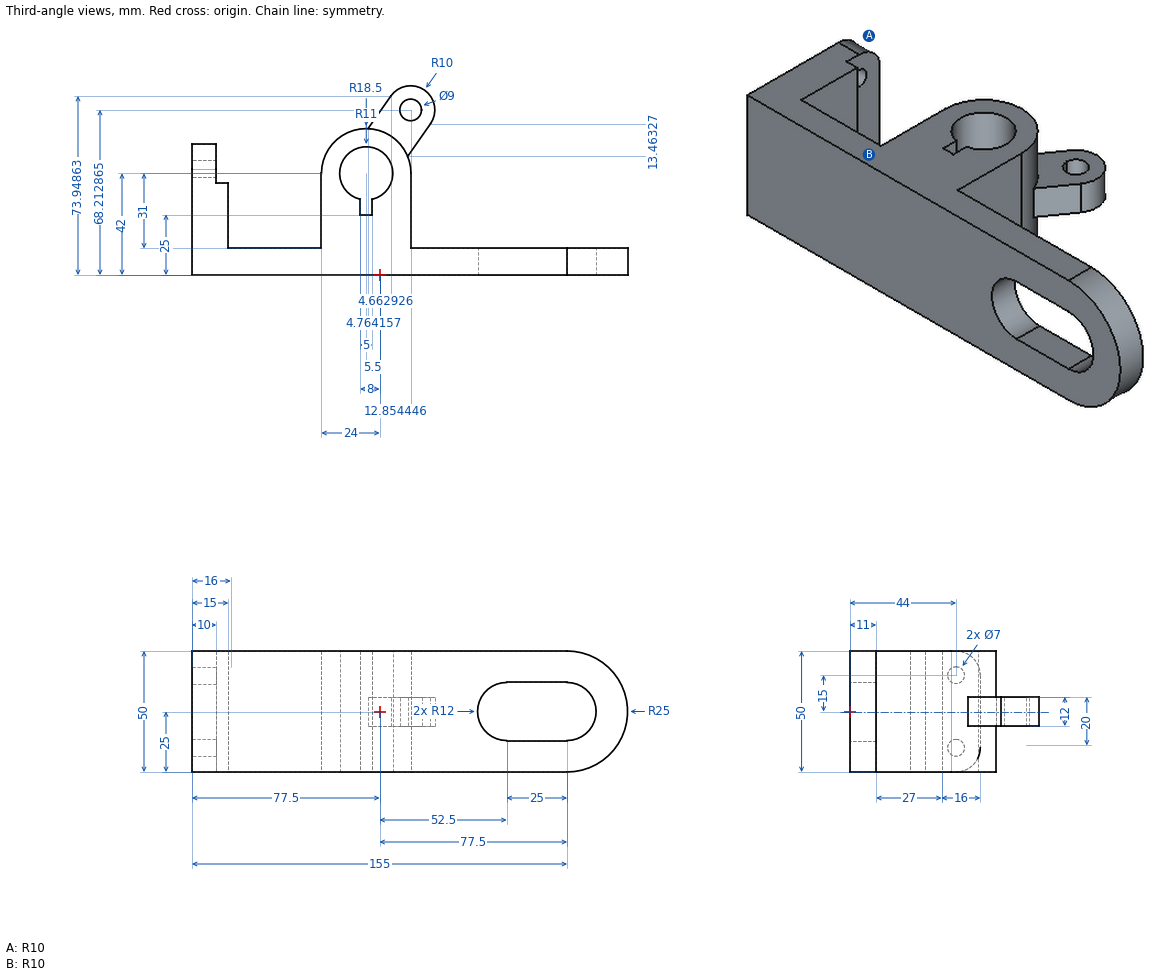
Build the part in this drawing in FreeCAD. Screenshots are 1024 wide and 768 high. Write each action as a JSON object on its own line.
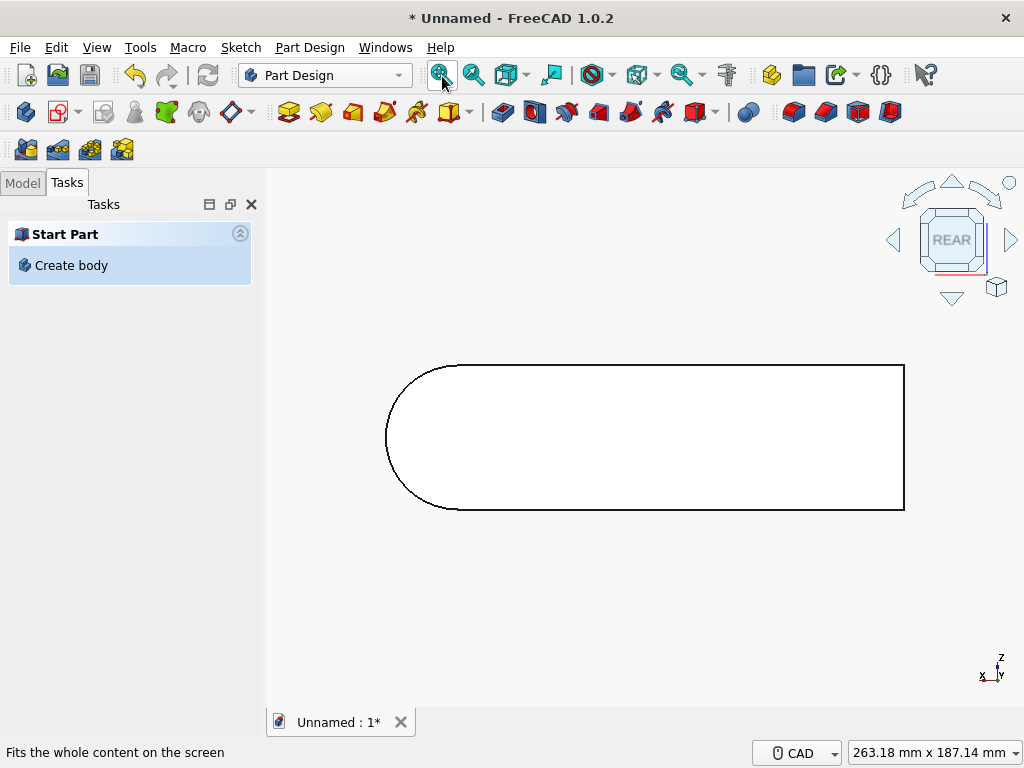
{"action": "left_click", "coordinate": [497, 436]}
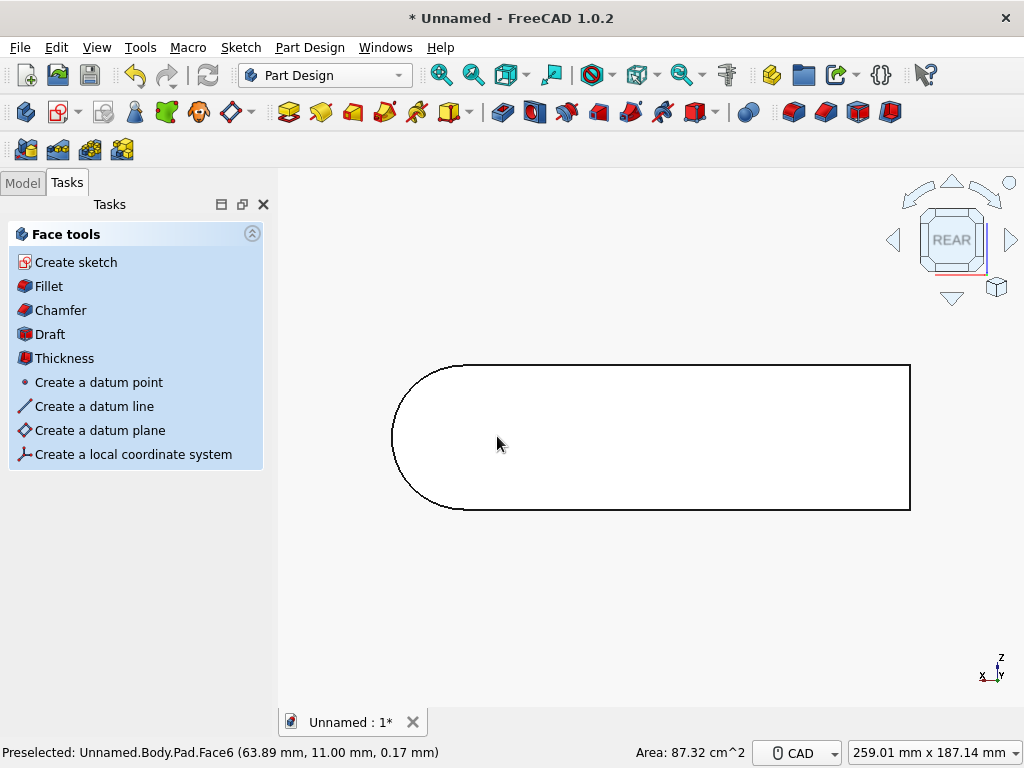
{"action": "left_click", "coordinate": [58, 112]}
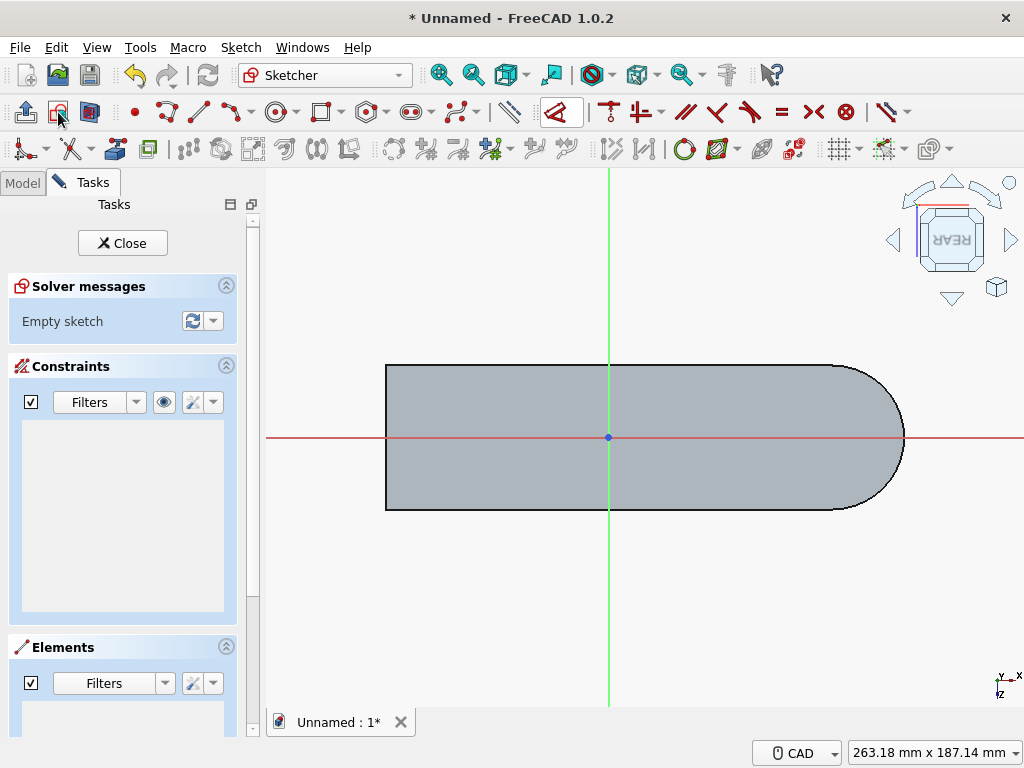
{"action": "scroll", "coordinate": [294, 437], "scroll_direction": "down", "scroll_amount": 1}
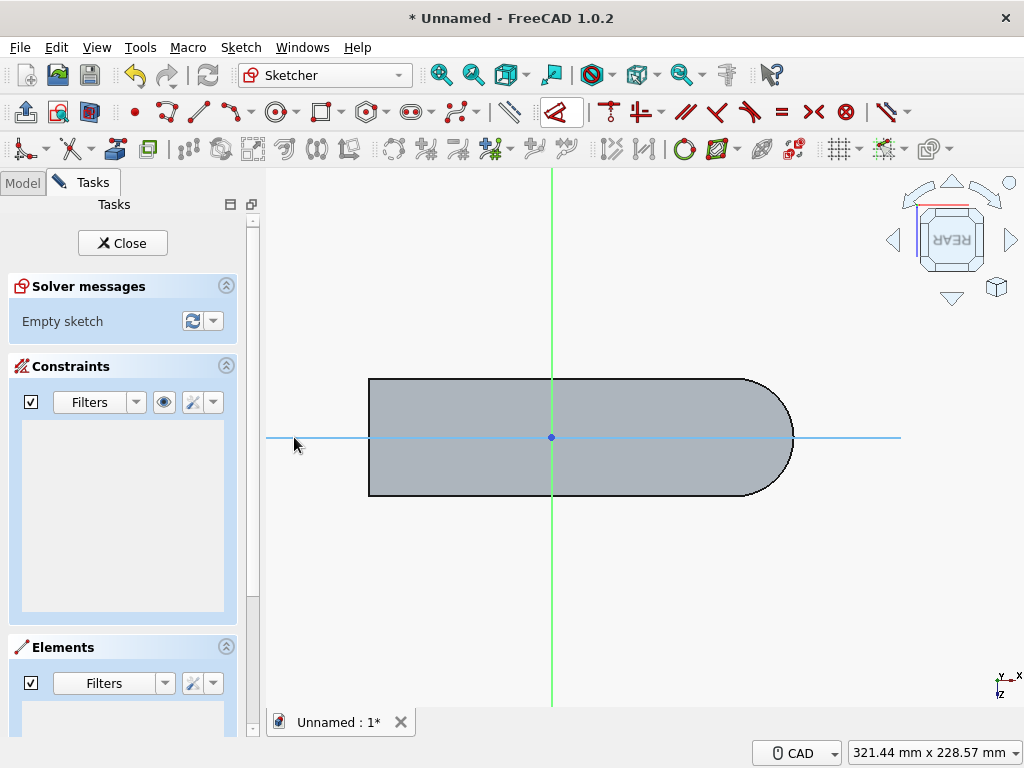
{"action": "scroll", "coordinate": [756, 438], "scroll_direction": "up", "scroll_amount": 3}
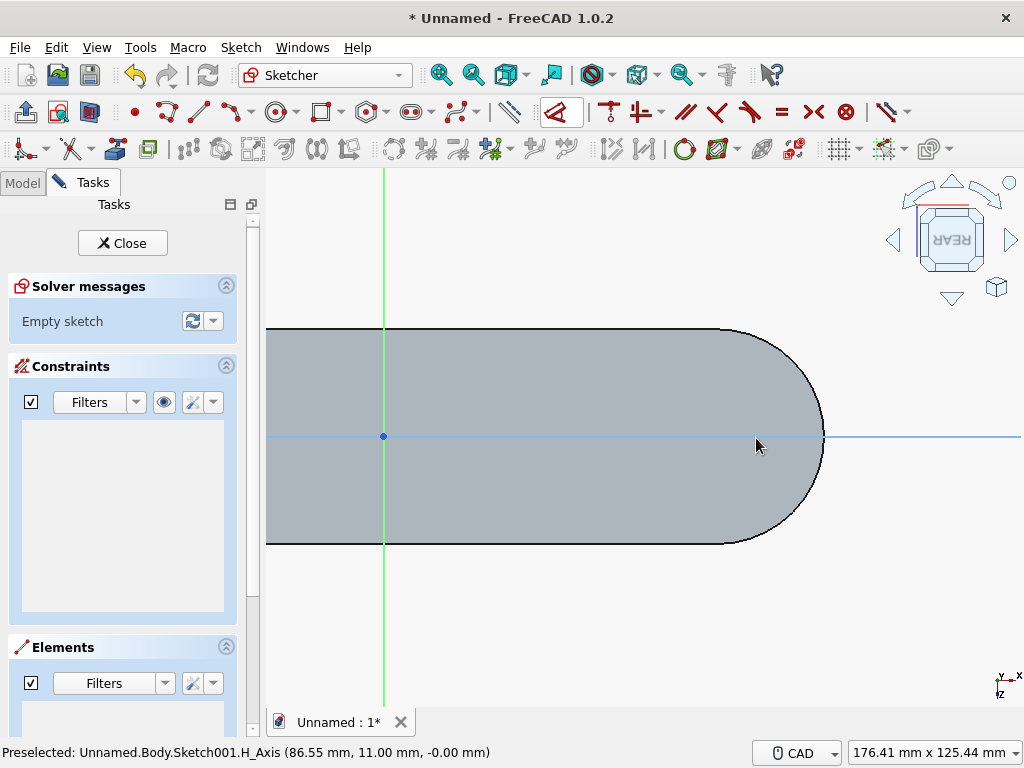
{"action": "left_click", "coordinate": [412, 112]}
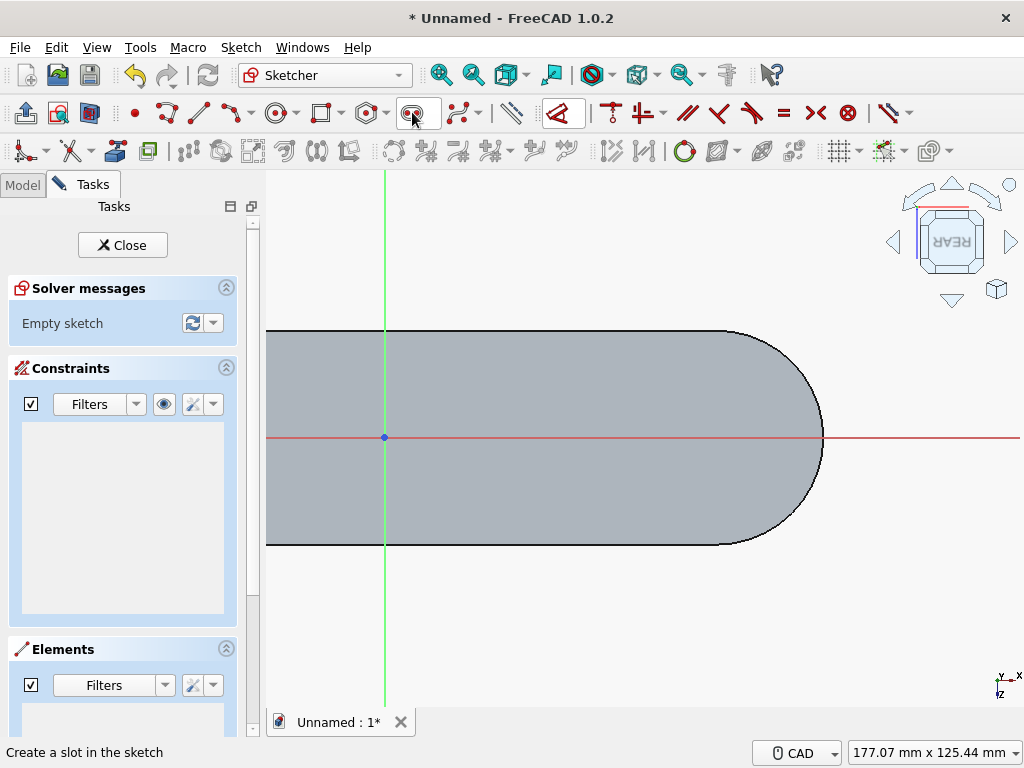
{"action": "left_click", "coordinate": [609, 438]}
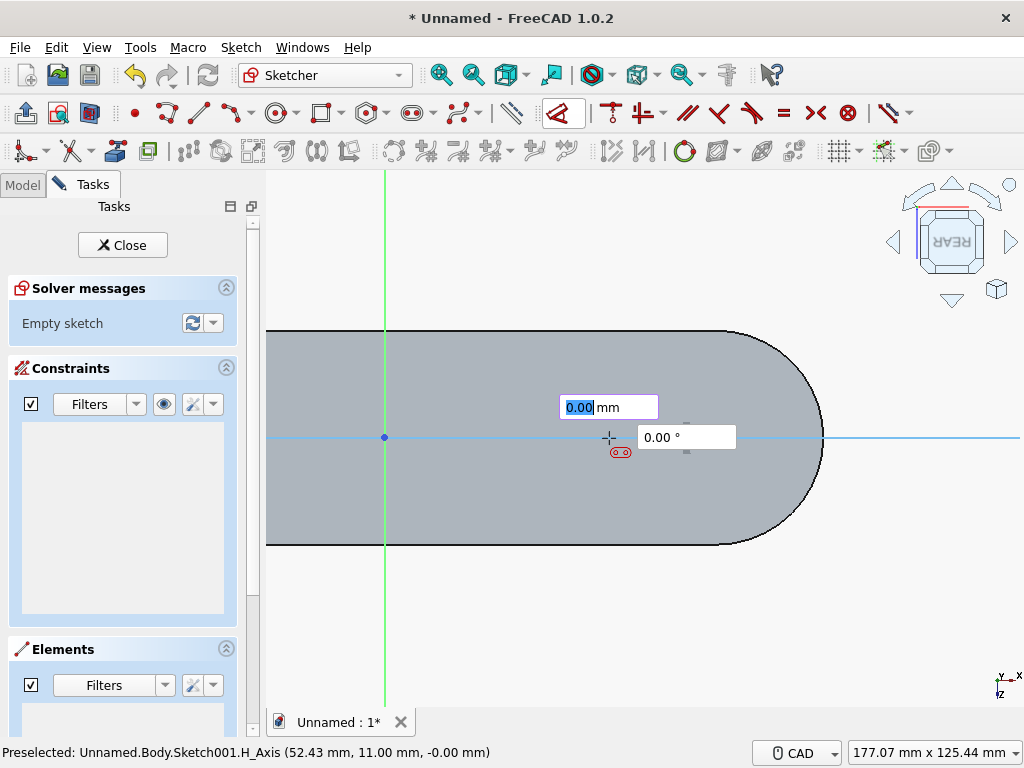
{"action": "left_click", "coordinate": [716, 429]}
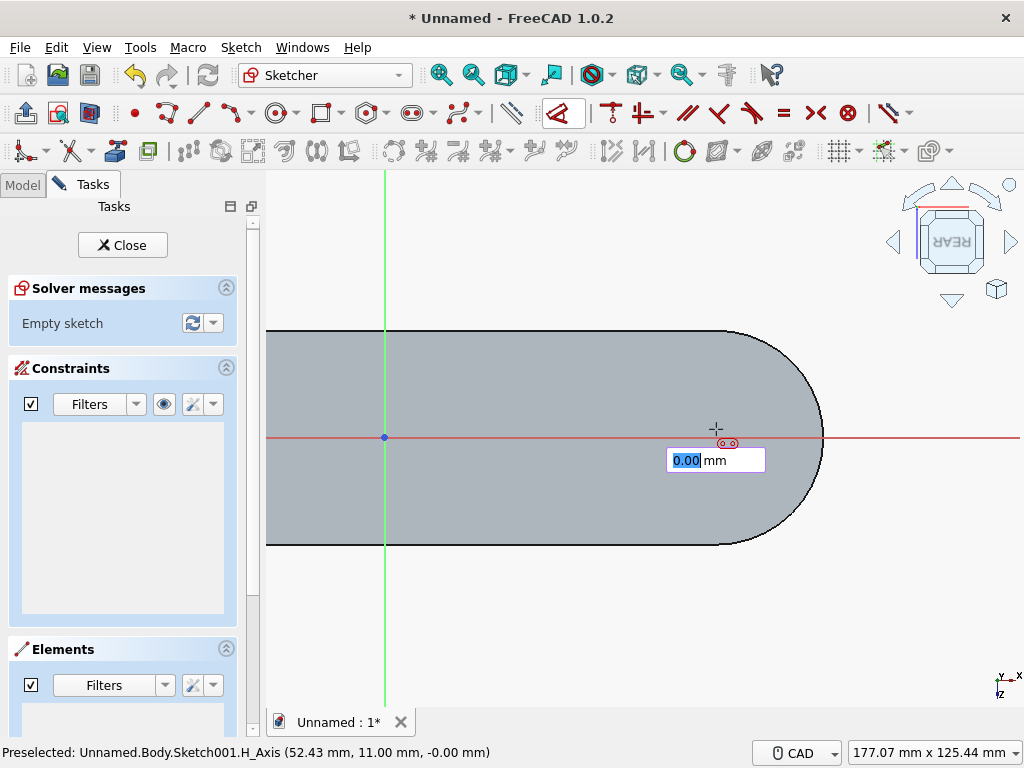
{"action": "left_click", "coordinate": [663, 386]}
{"action": "key", "text": "Escape"}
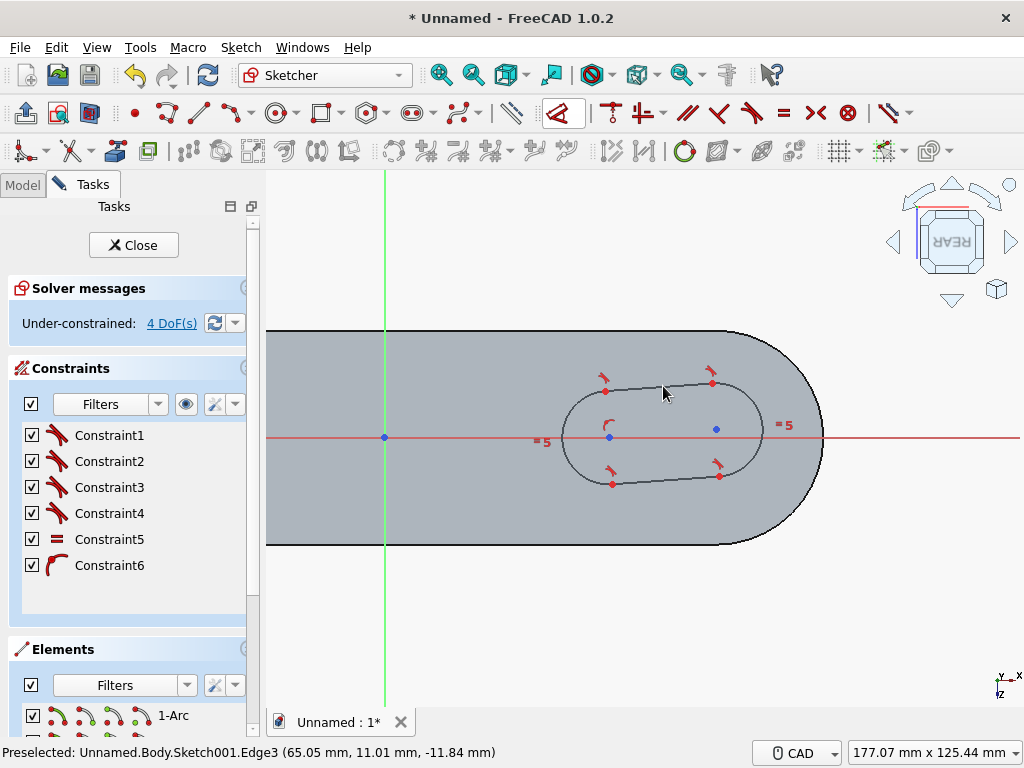
{"action": "left_click", "coordinate": [638, 389]}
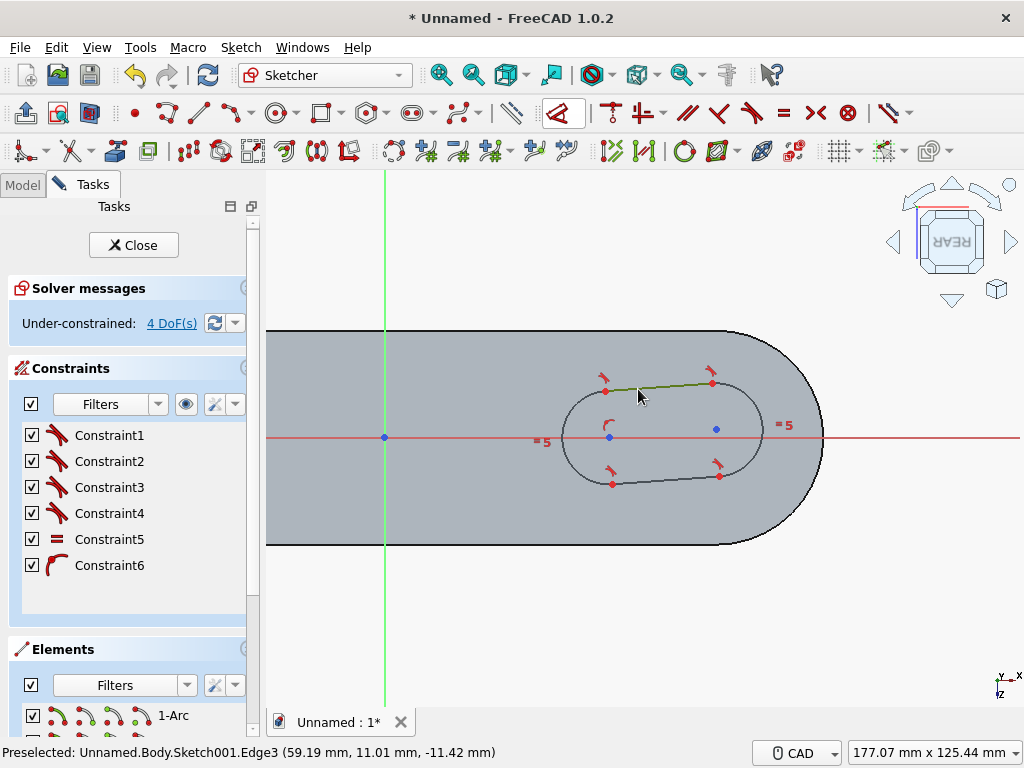
{"action": "left_click", "coordinate": [666, 114]}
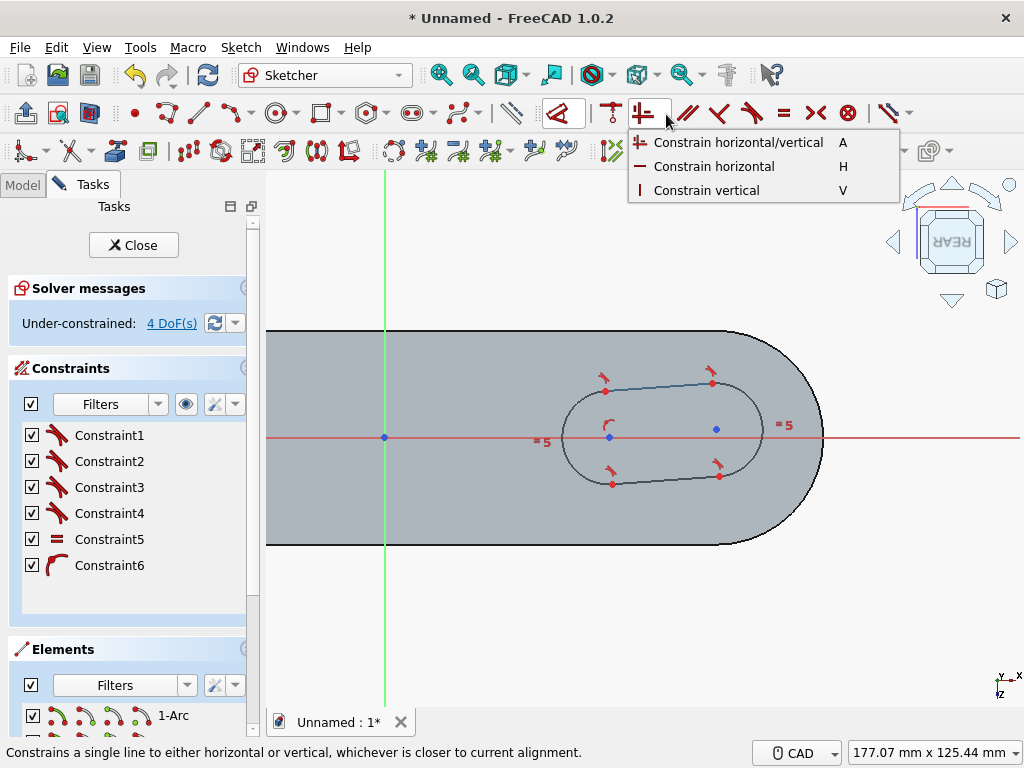
{"action": "left_click", "coordinate": [764, 166]}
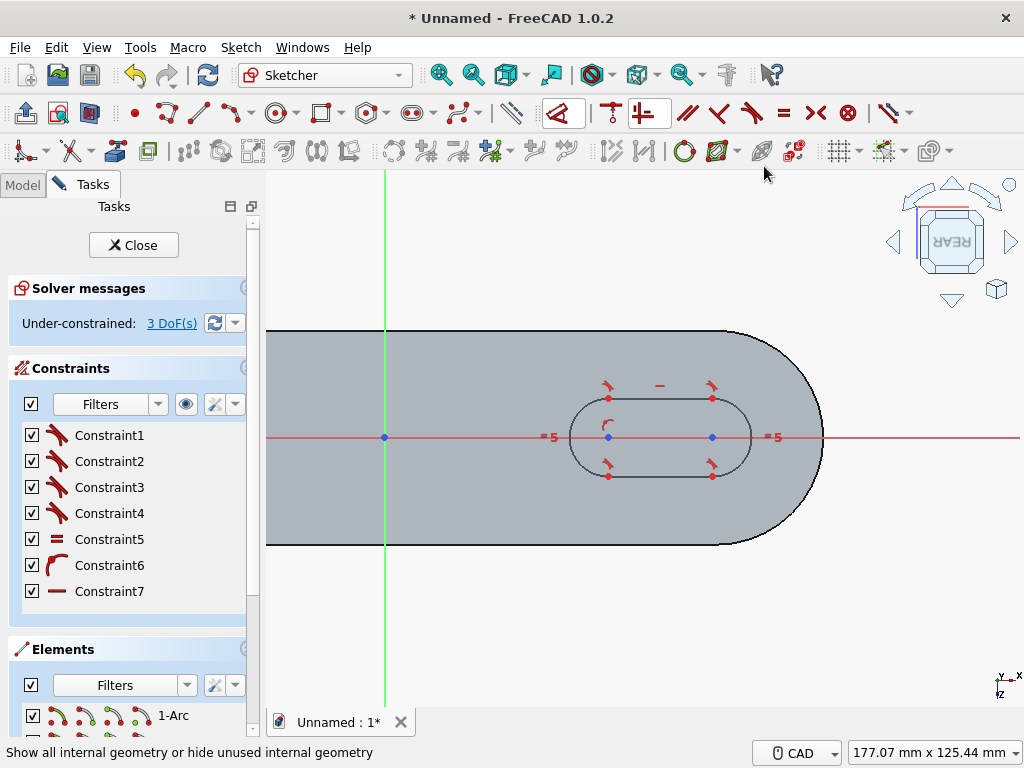
{"action": "left_click", "coordinate": [577, 415]}